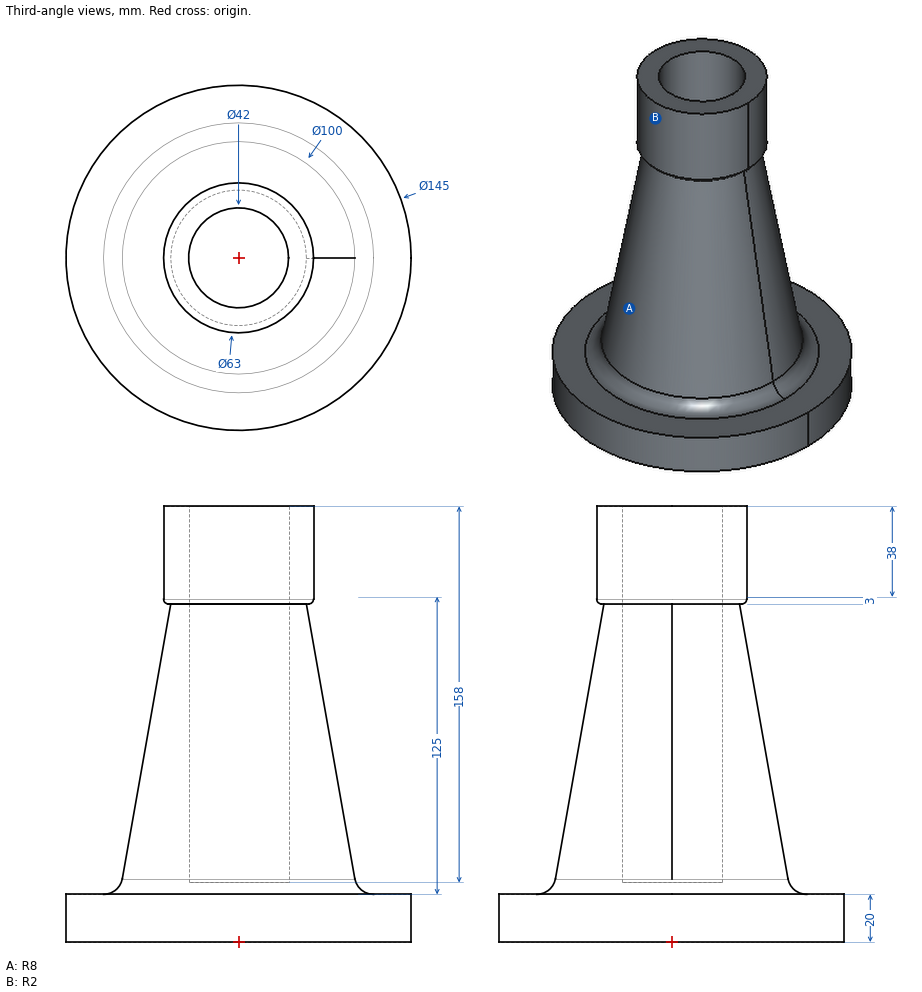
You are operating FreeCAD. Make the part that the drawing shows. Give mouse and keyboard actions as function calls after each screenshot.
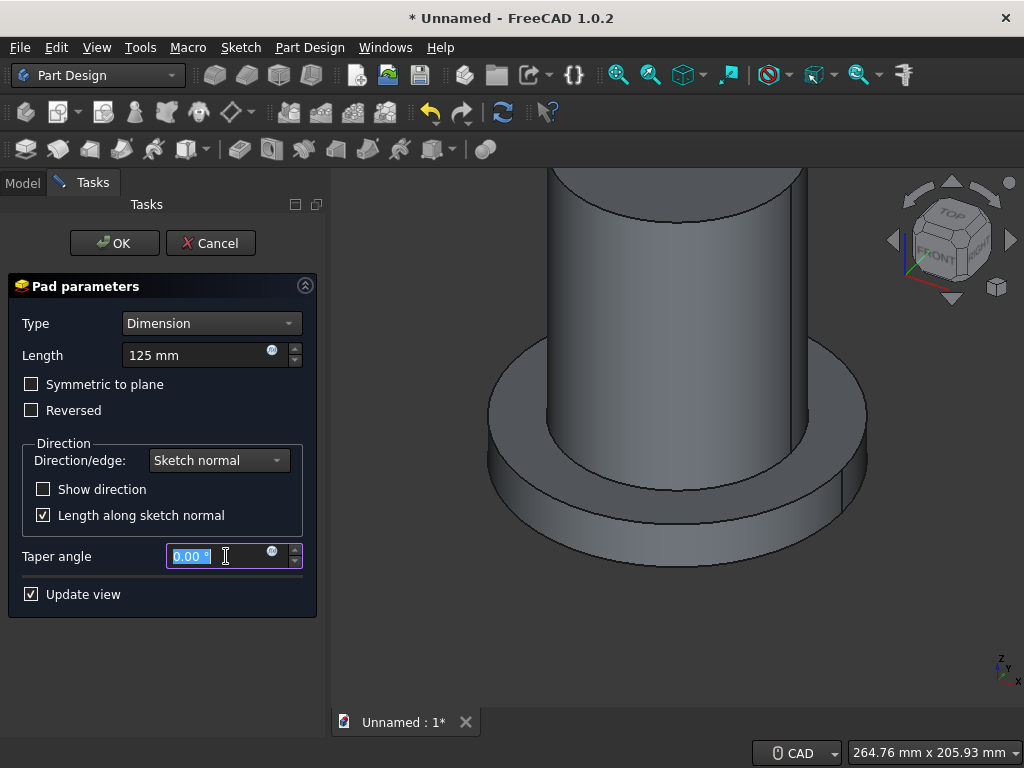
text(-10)
key(Tab)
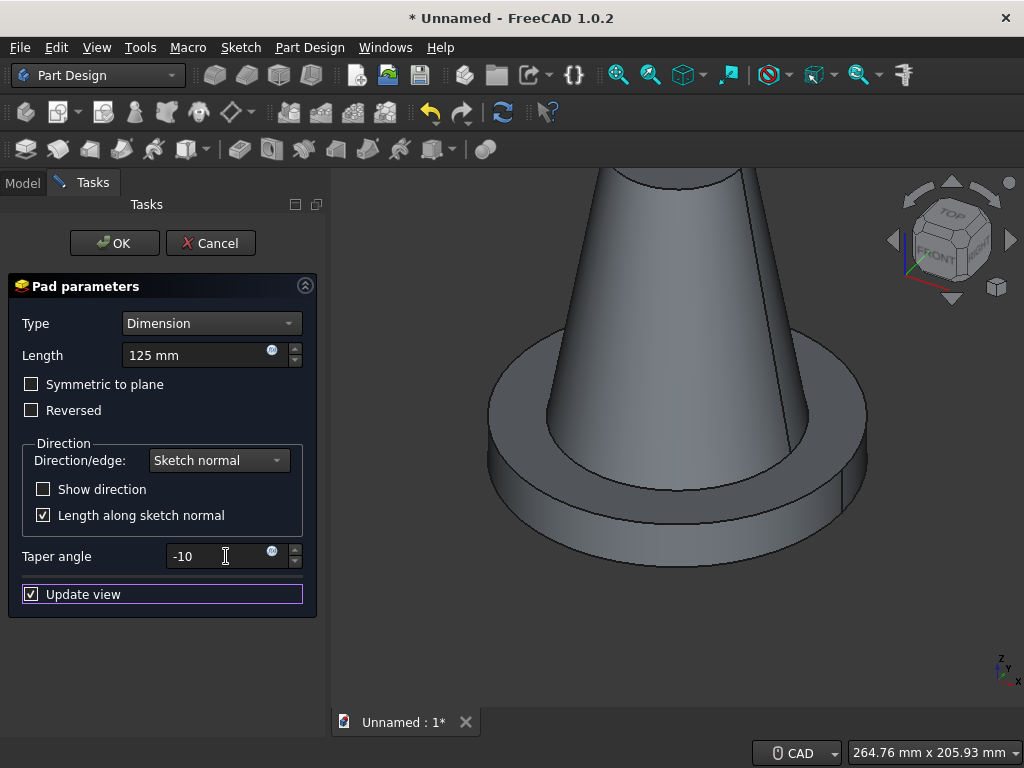
click(115, 243)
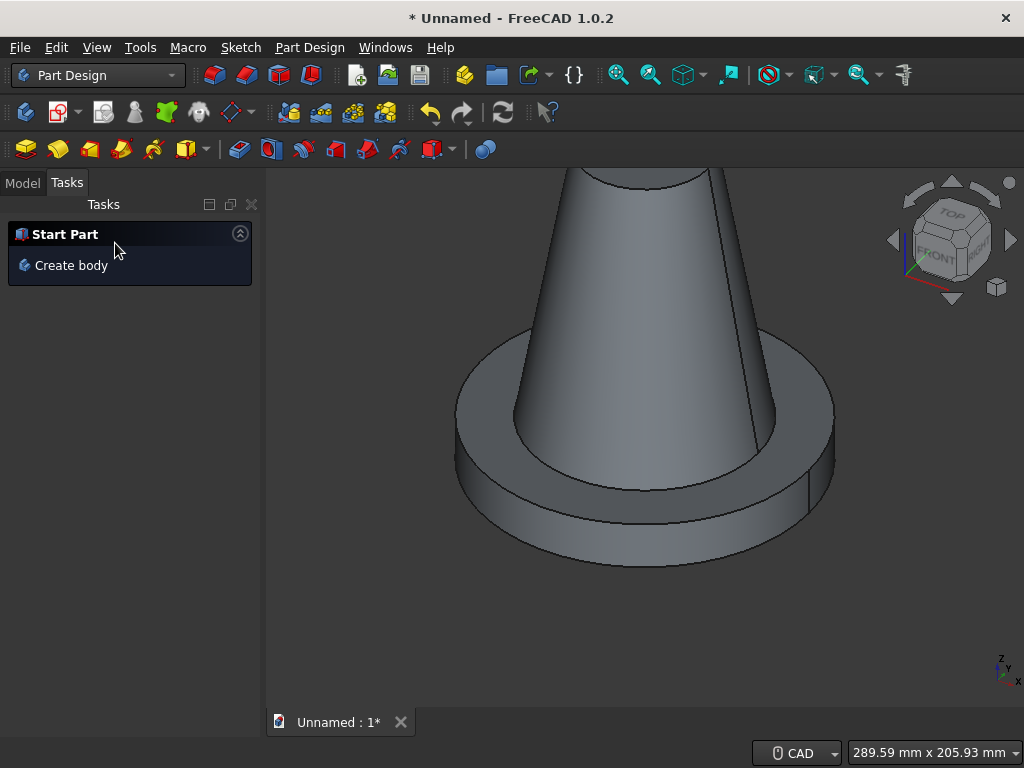
key(v)
key(f)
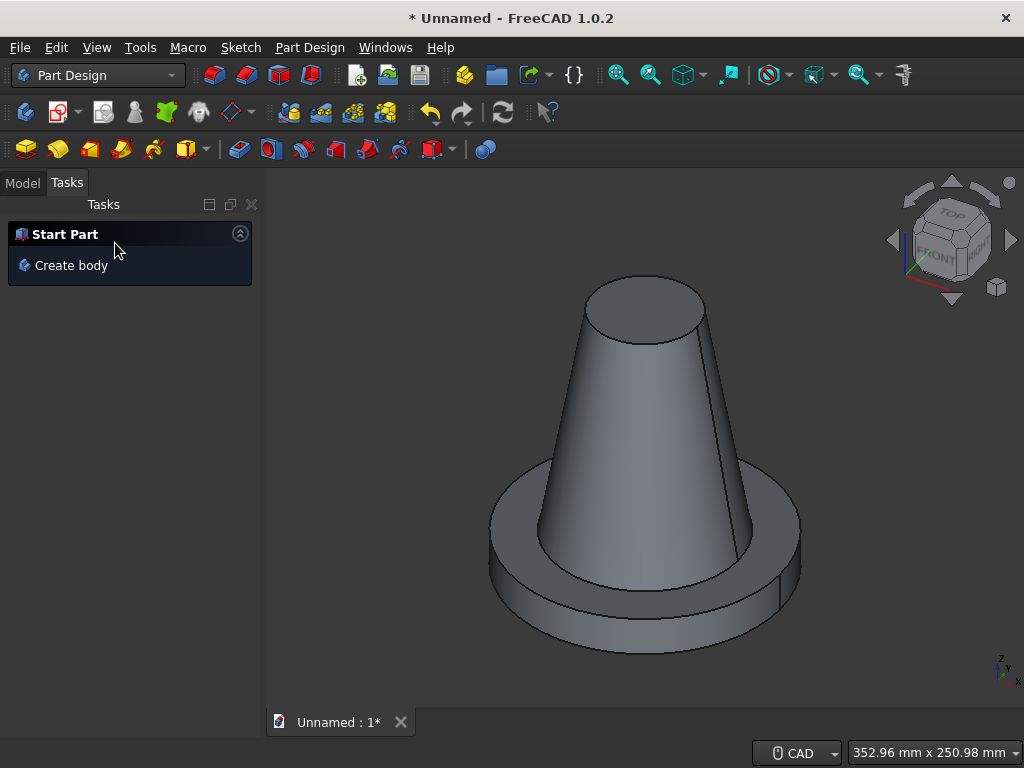
click(645, 309)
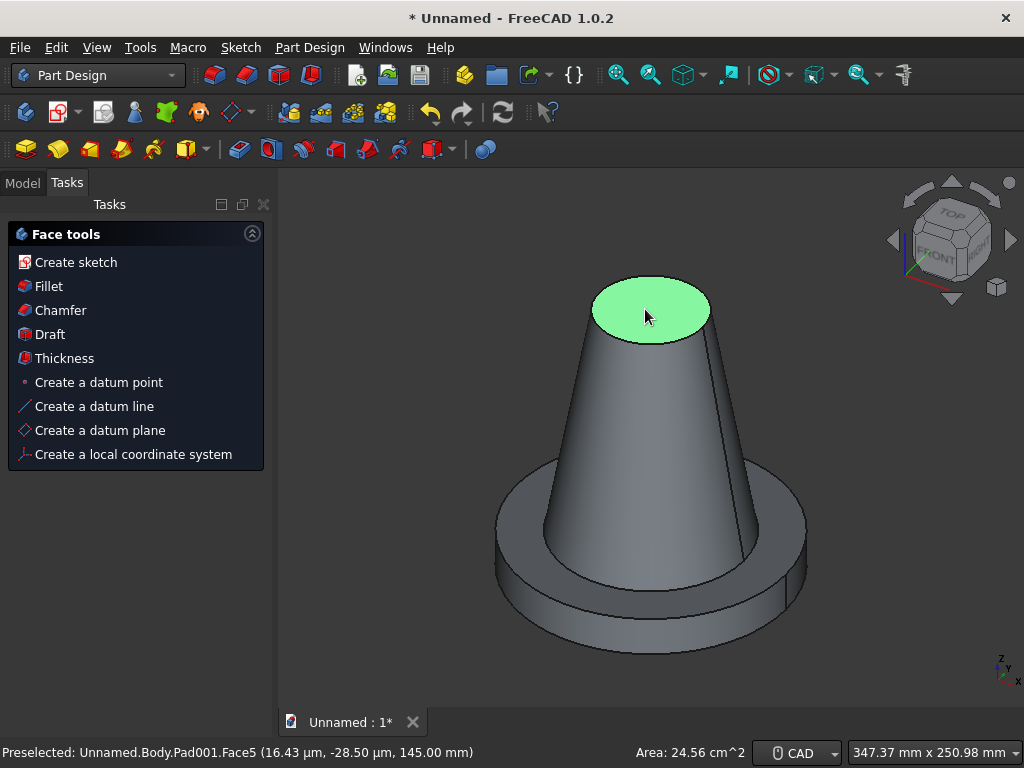
click(58, 112)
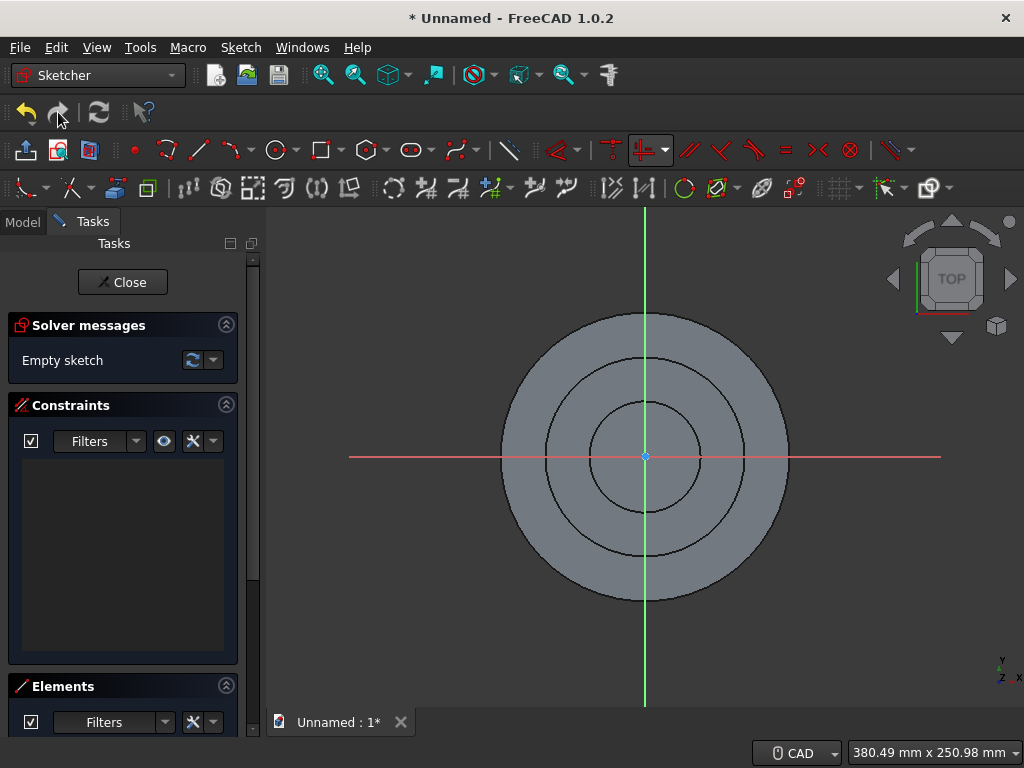
scroll(685, 457, up, 5)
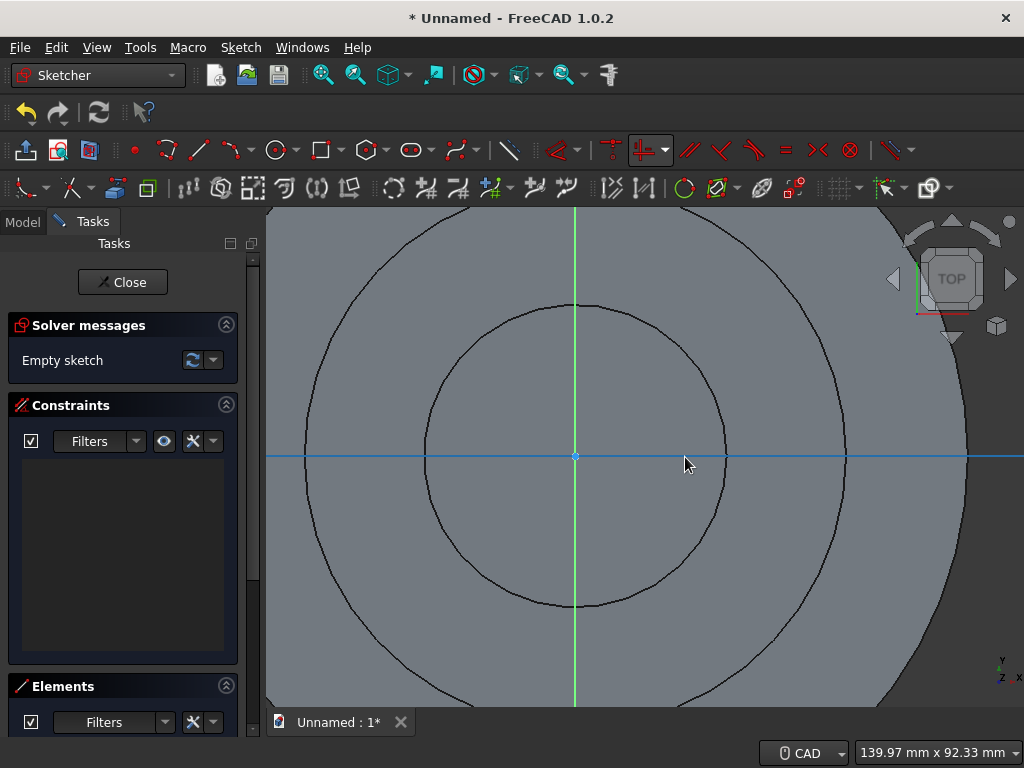
key(g)
key(c)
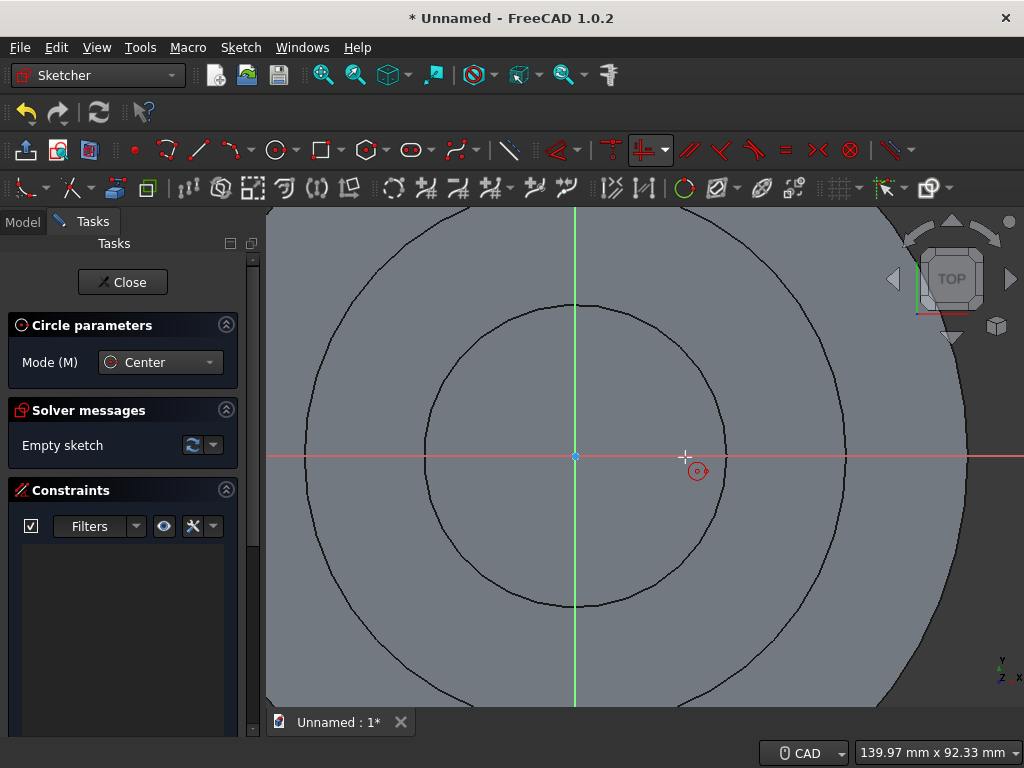
click(575, 456)
click(696, 336)
key(Escape)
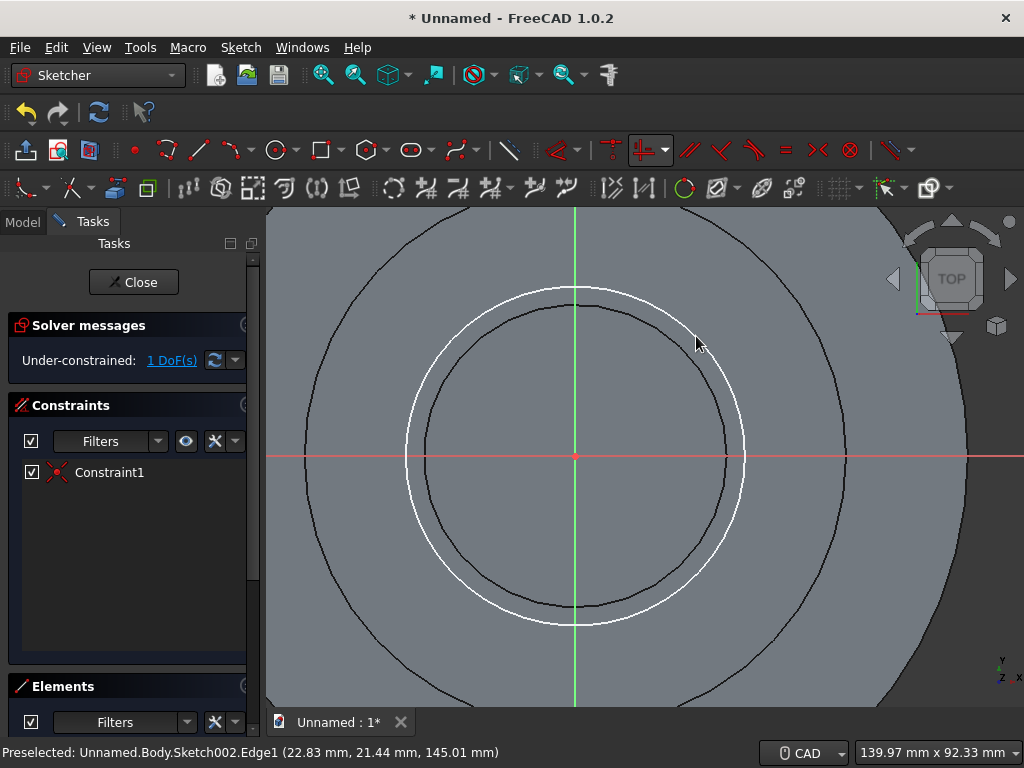
key(d)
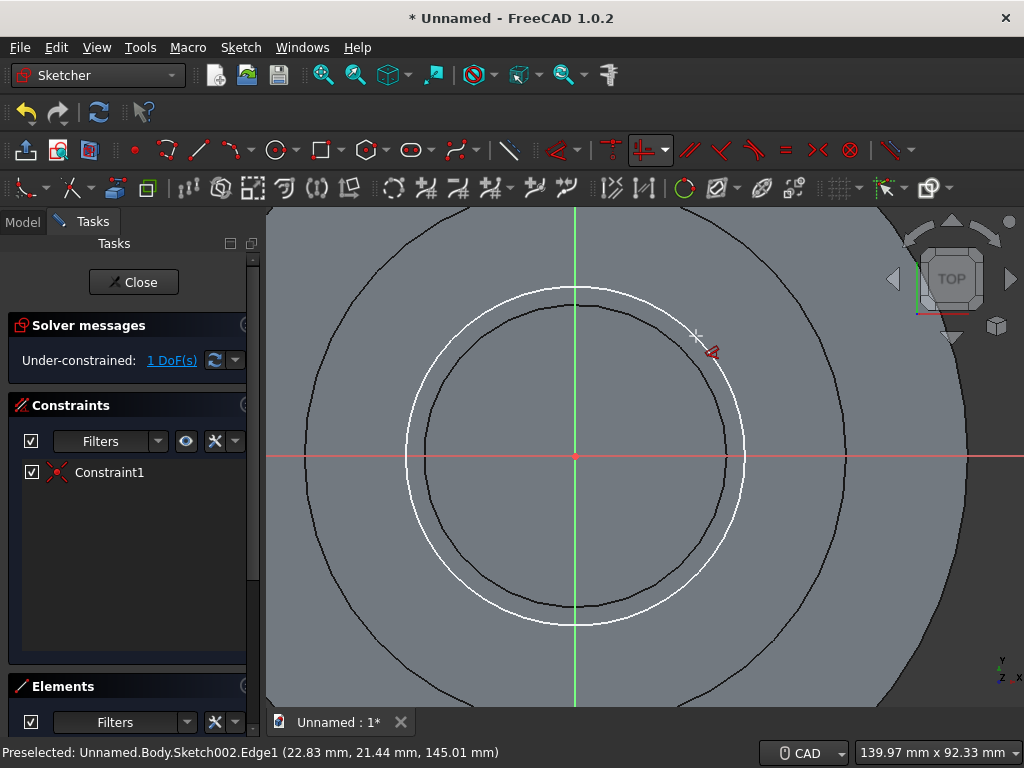
click(695, 336)
click(718, 313)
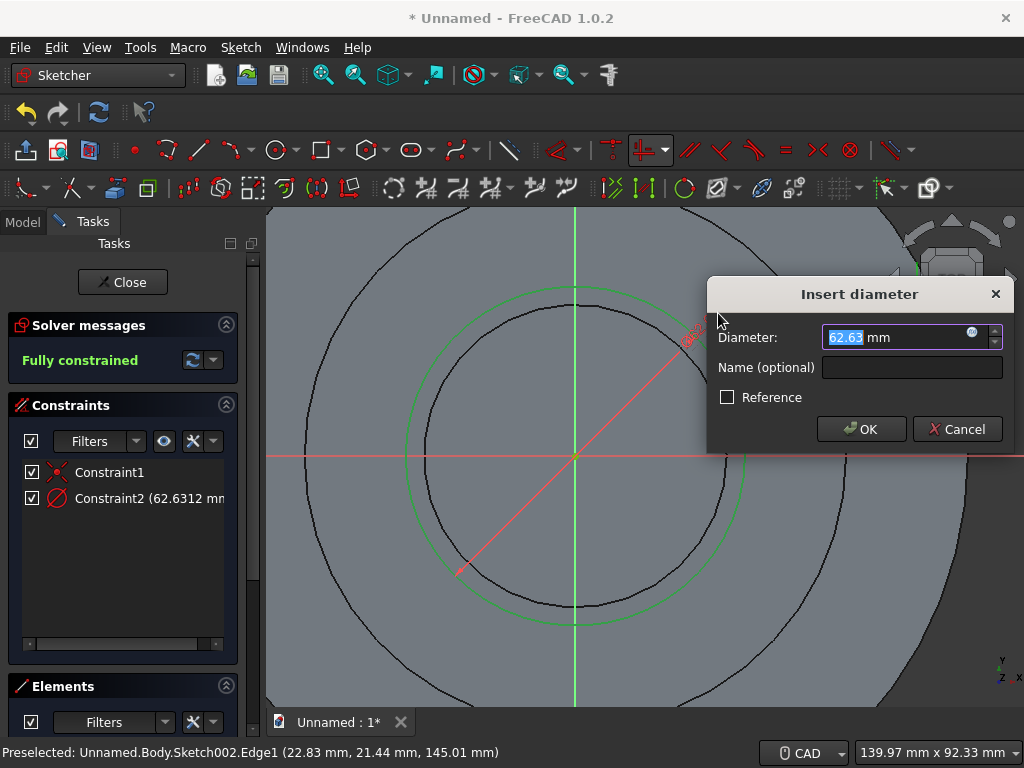
text(63)
key(Return)
key(Escape)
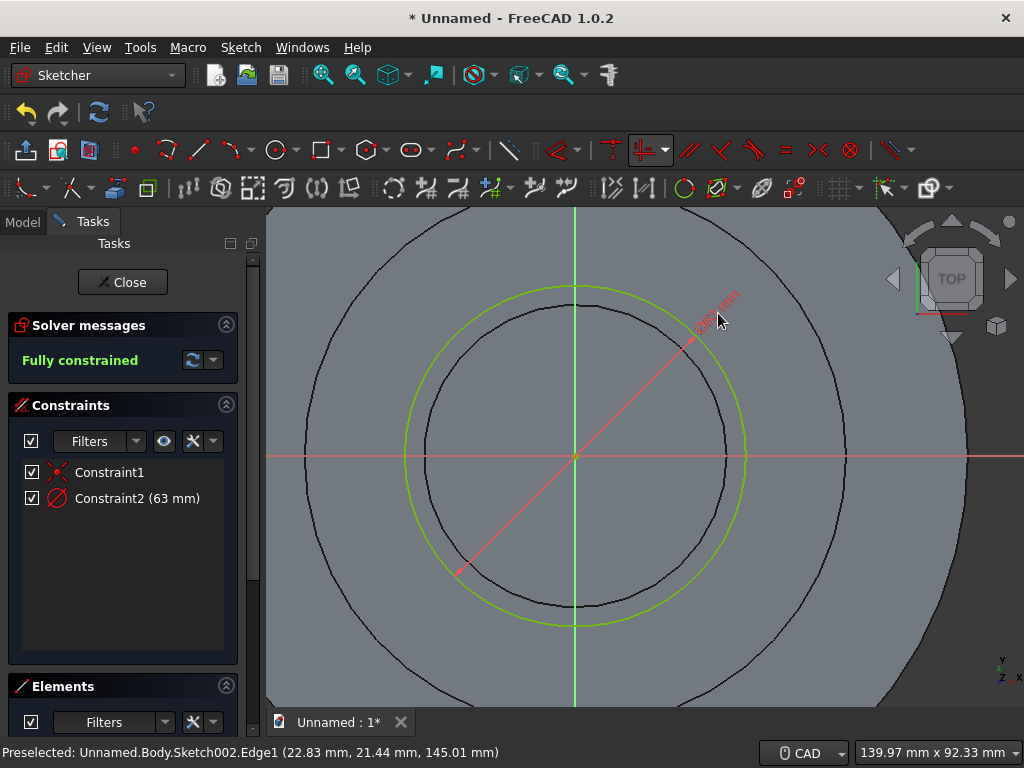
click(123, 282)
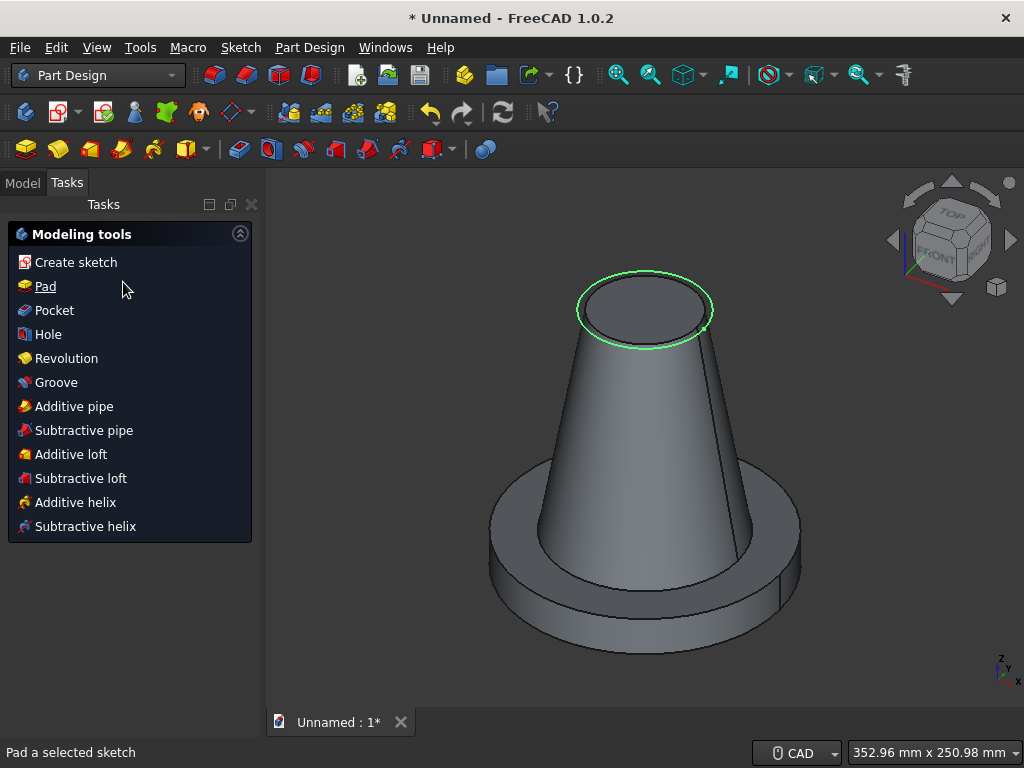
click(26, 150)